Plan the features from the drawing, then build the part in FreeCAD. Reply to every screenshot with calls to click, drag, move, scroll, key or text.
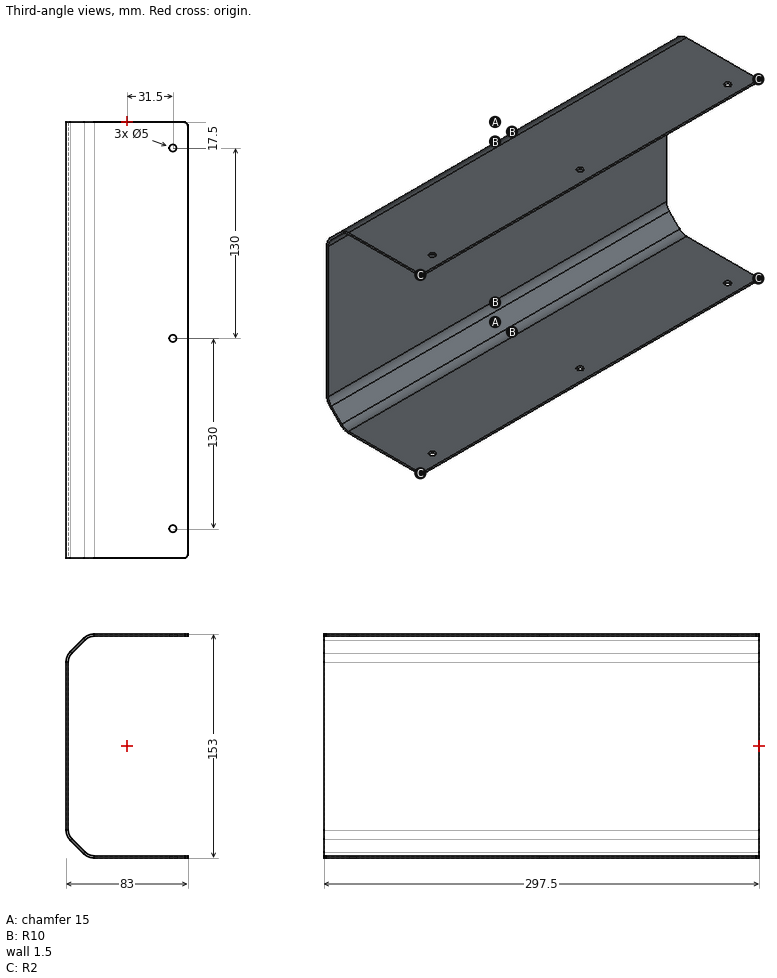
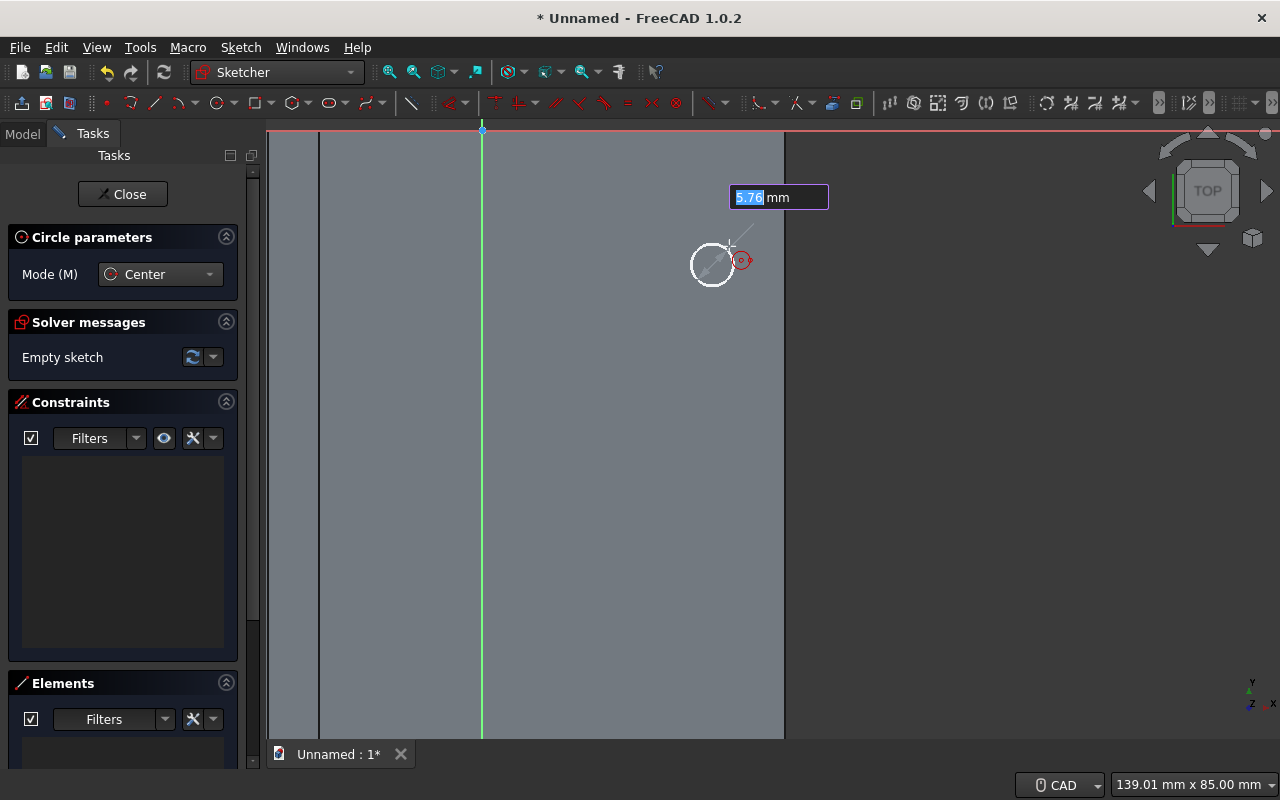
click(725, 245)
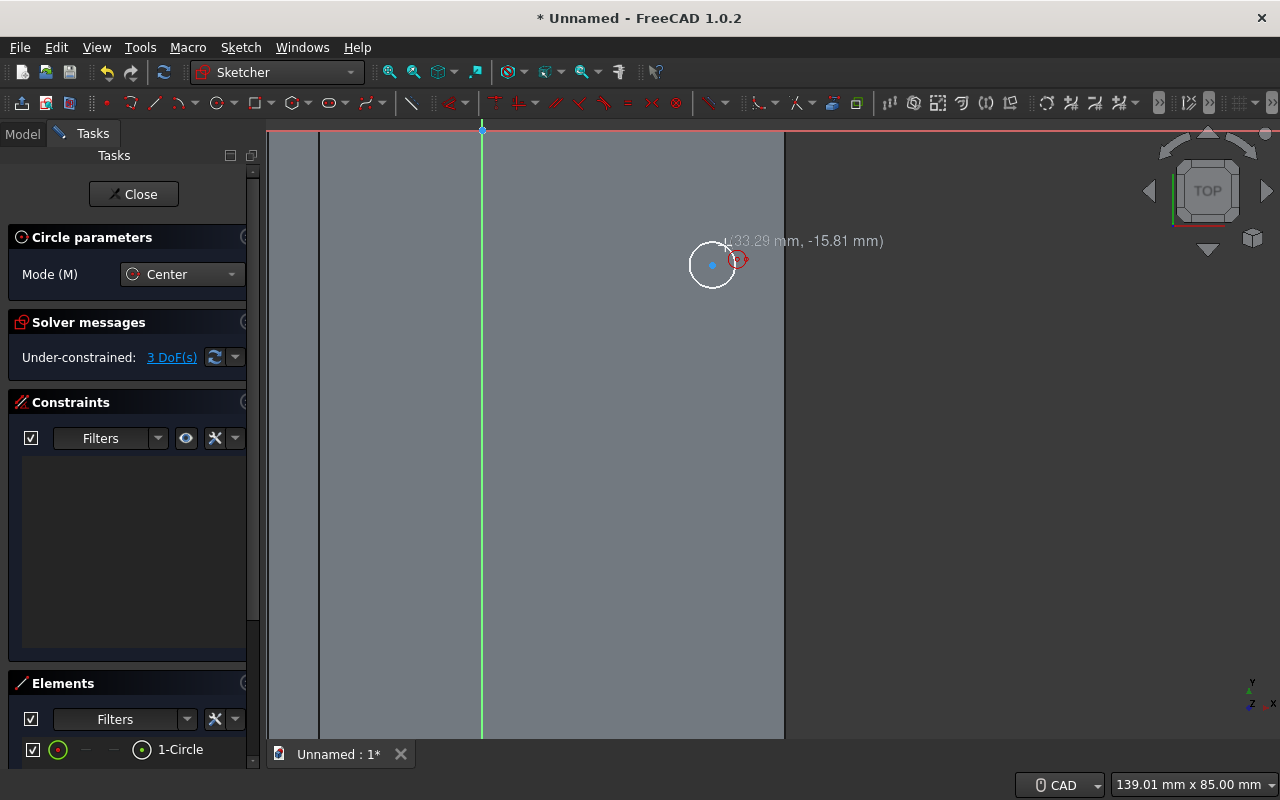
scroll(729, 246, down, 8)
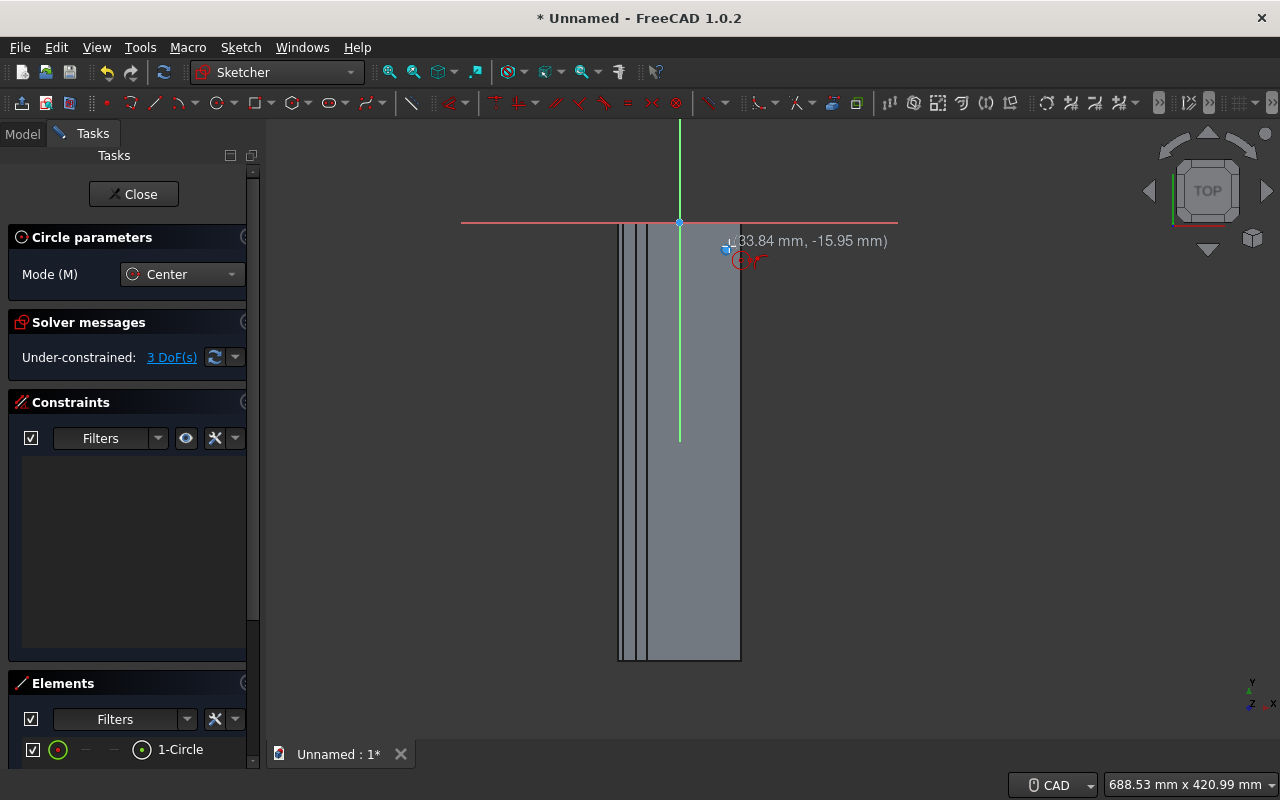
scroll(726, 440, up, 10)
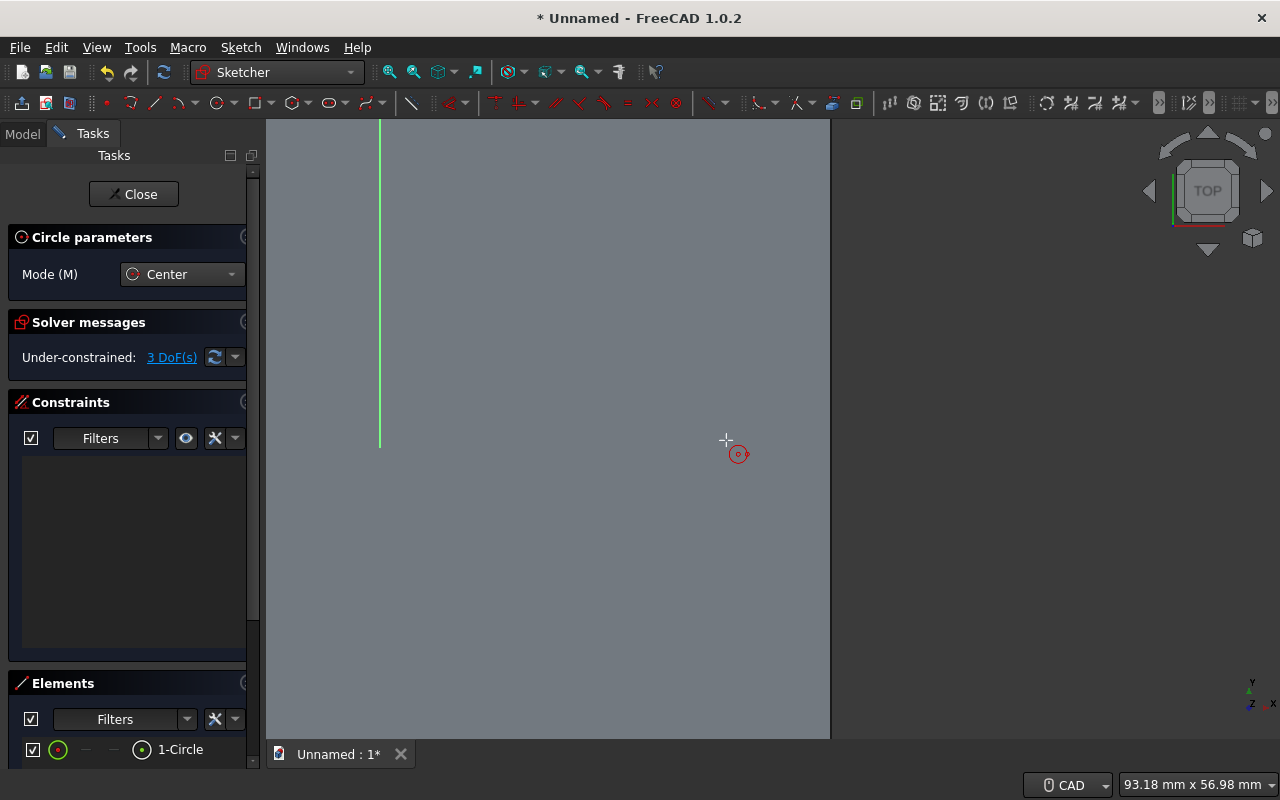
scroll(726, 440, down, 10)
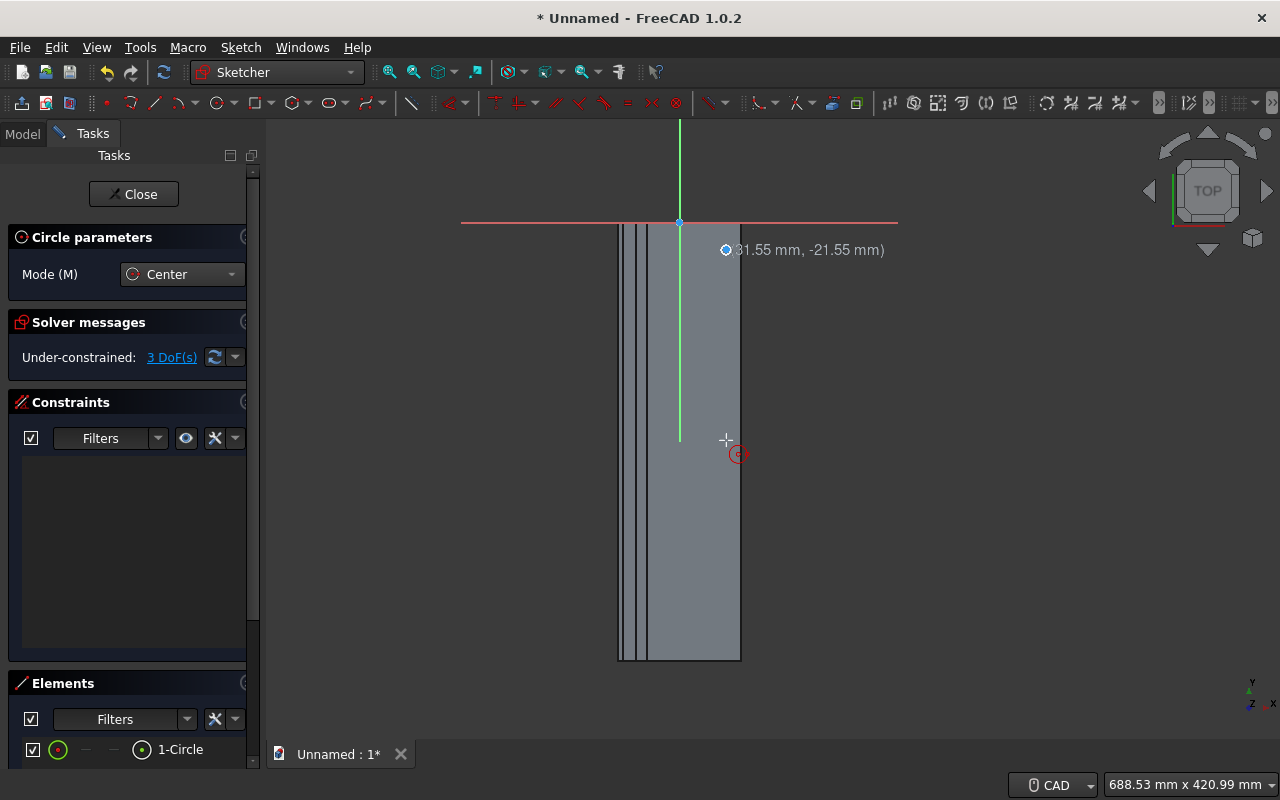
click(726, 440)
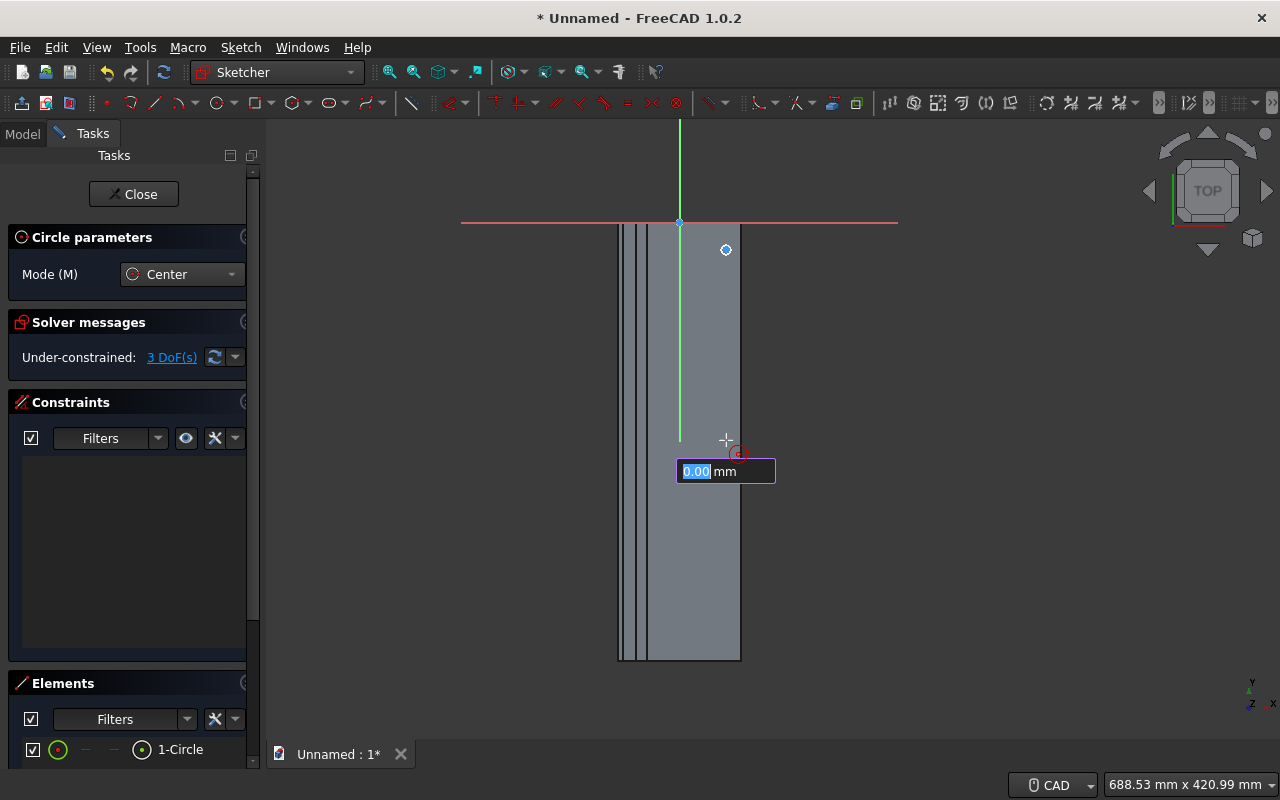
scroll(729, 437, up, 8)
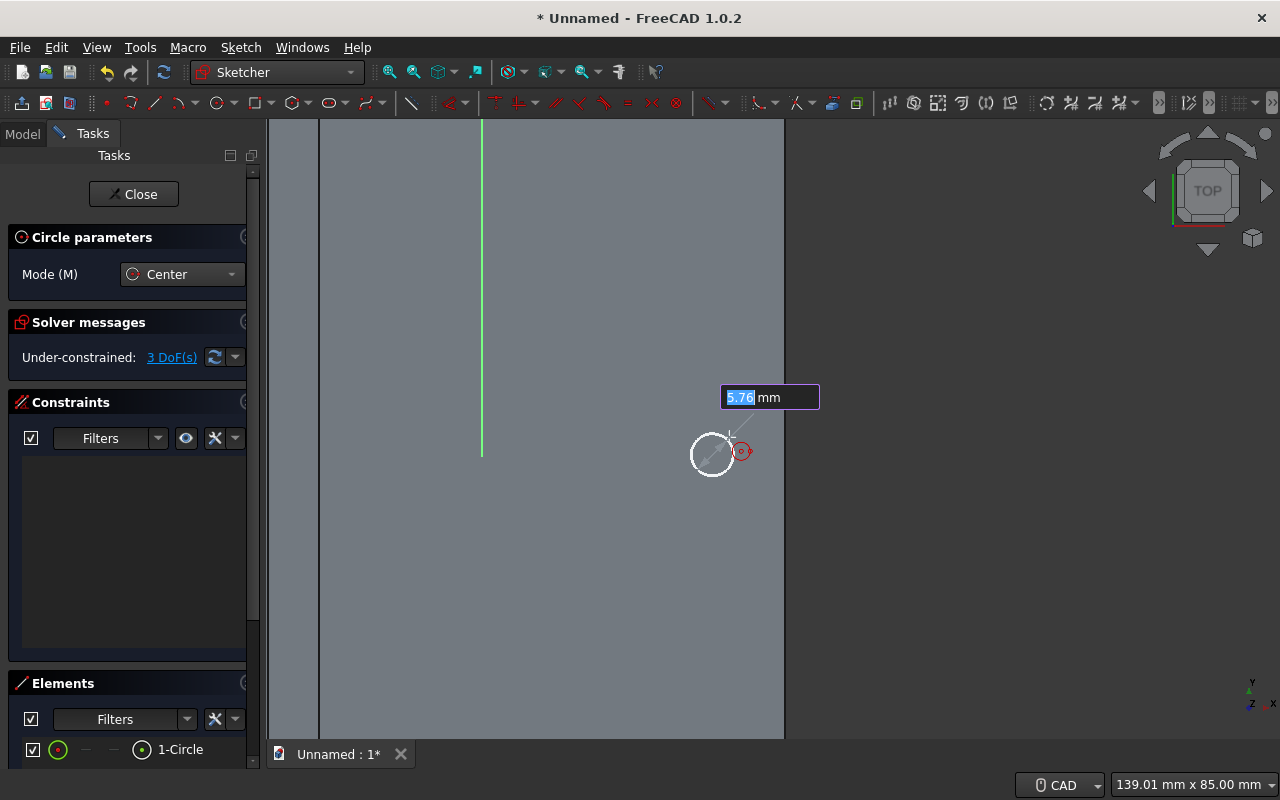
click(725, 437)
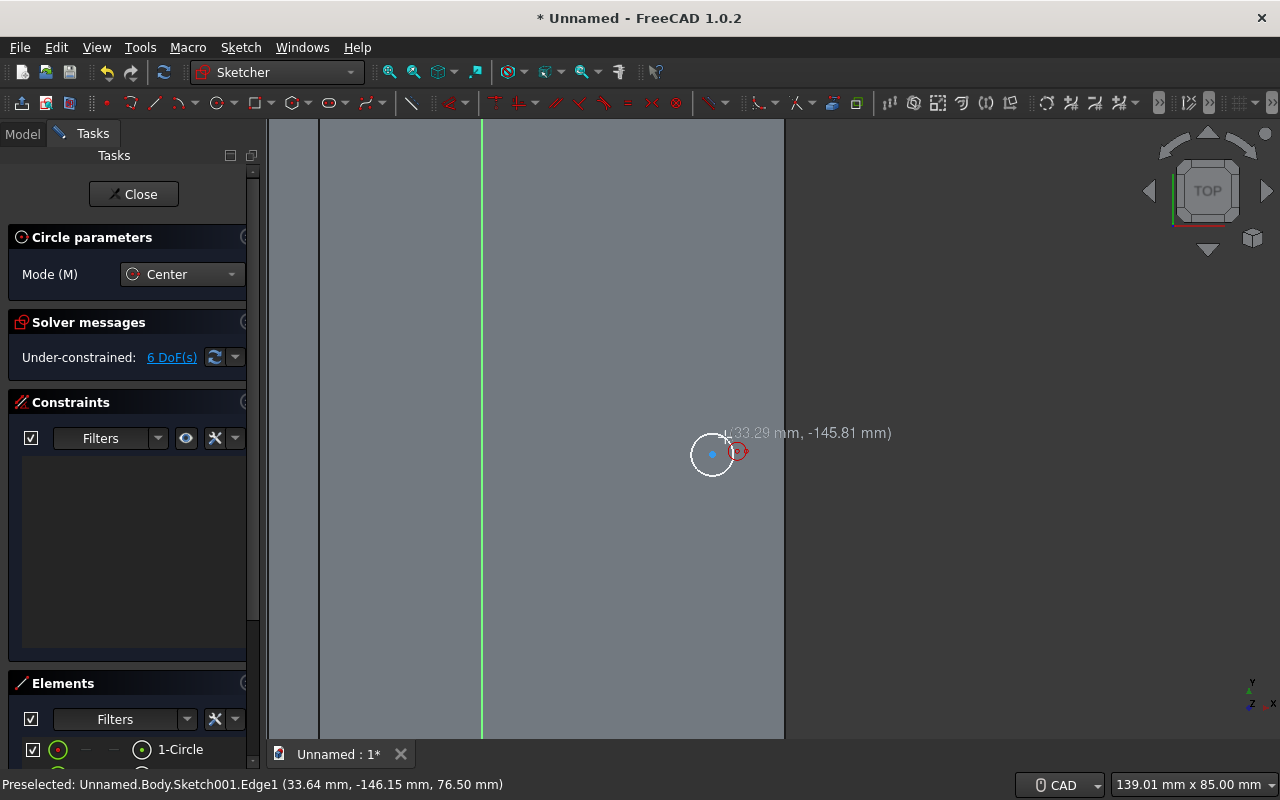
scroll(729, 437, down, 8)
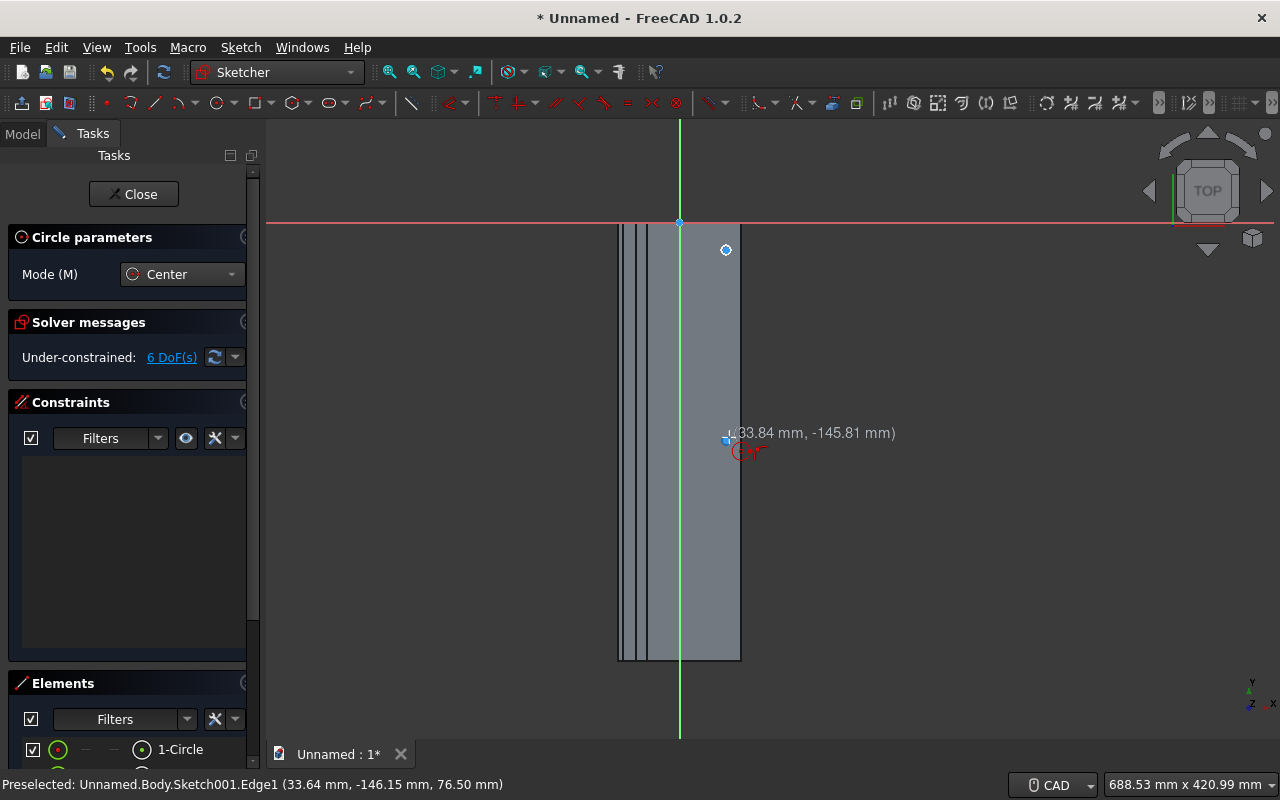
scroll(726, 632, up, 10)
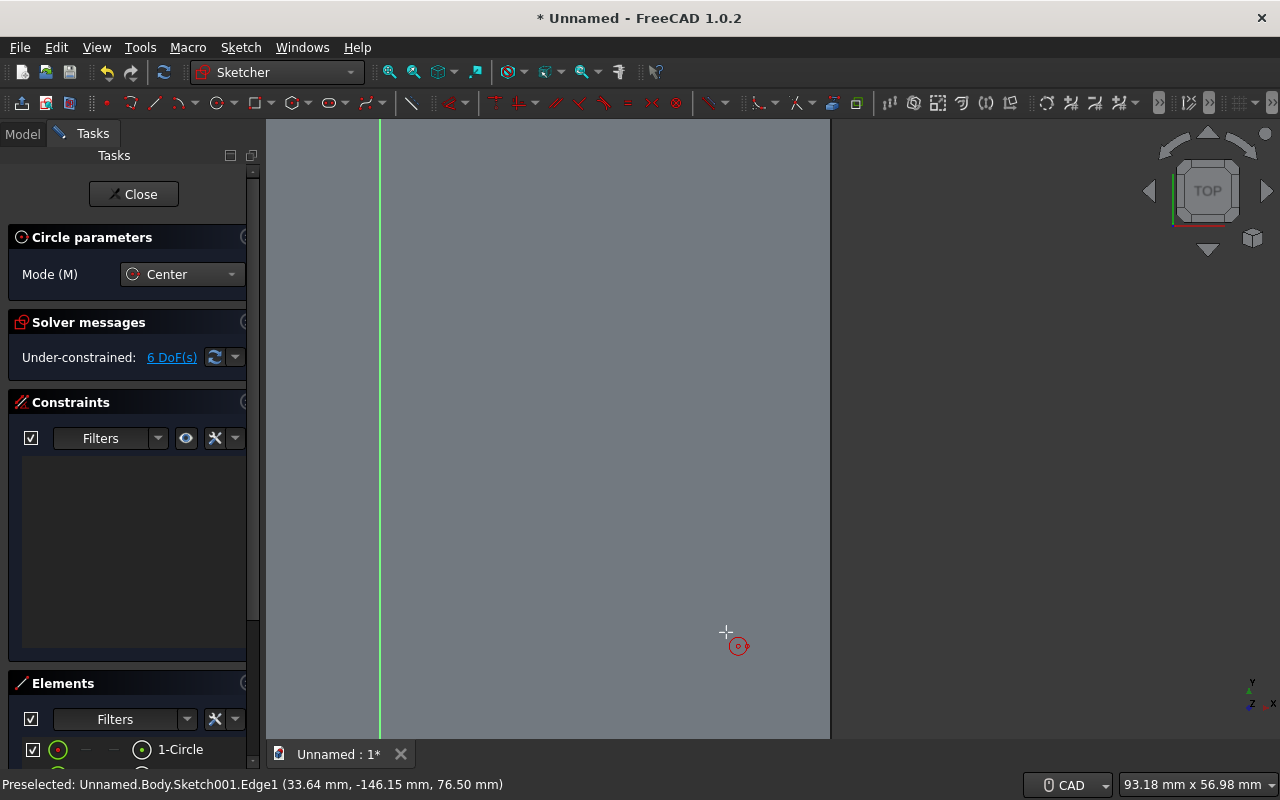
scroll(726, 633, down, 10)